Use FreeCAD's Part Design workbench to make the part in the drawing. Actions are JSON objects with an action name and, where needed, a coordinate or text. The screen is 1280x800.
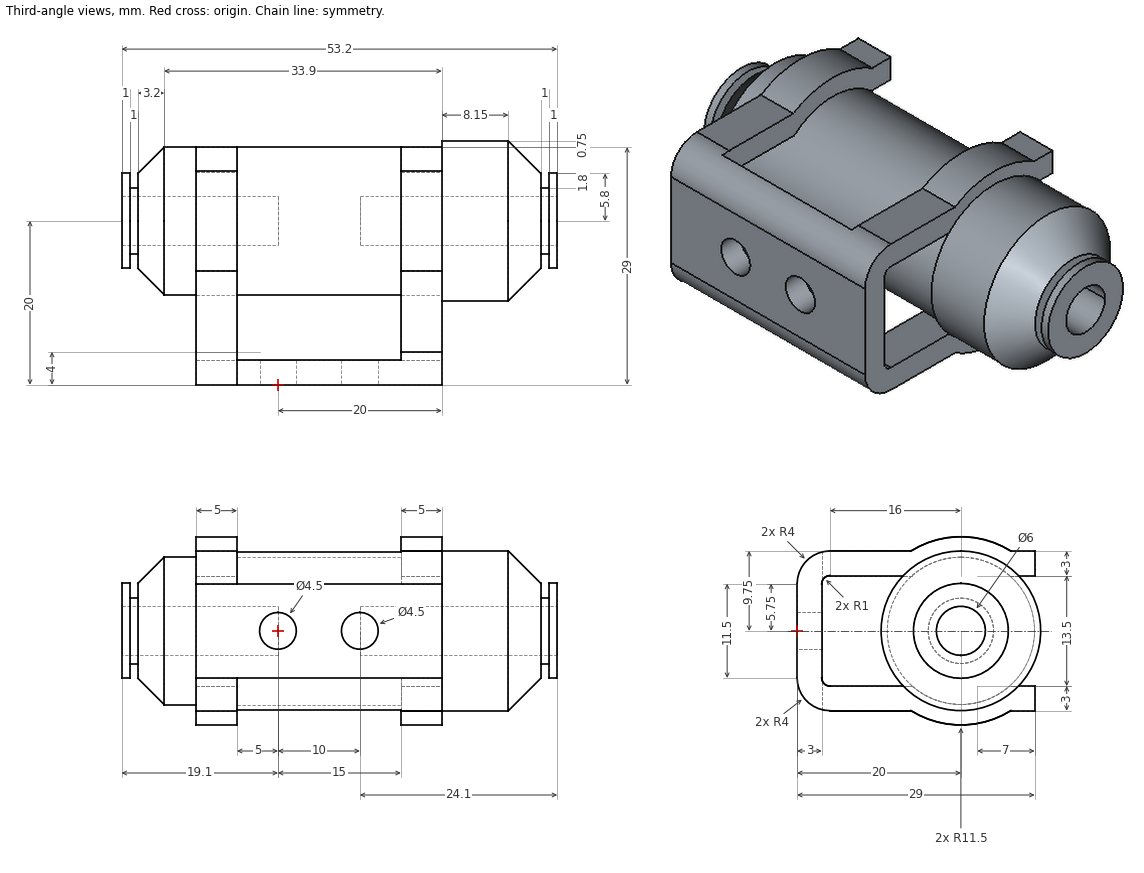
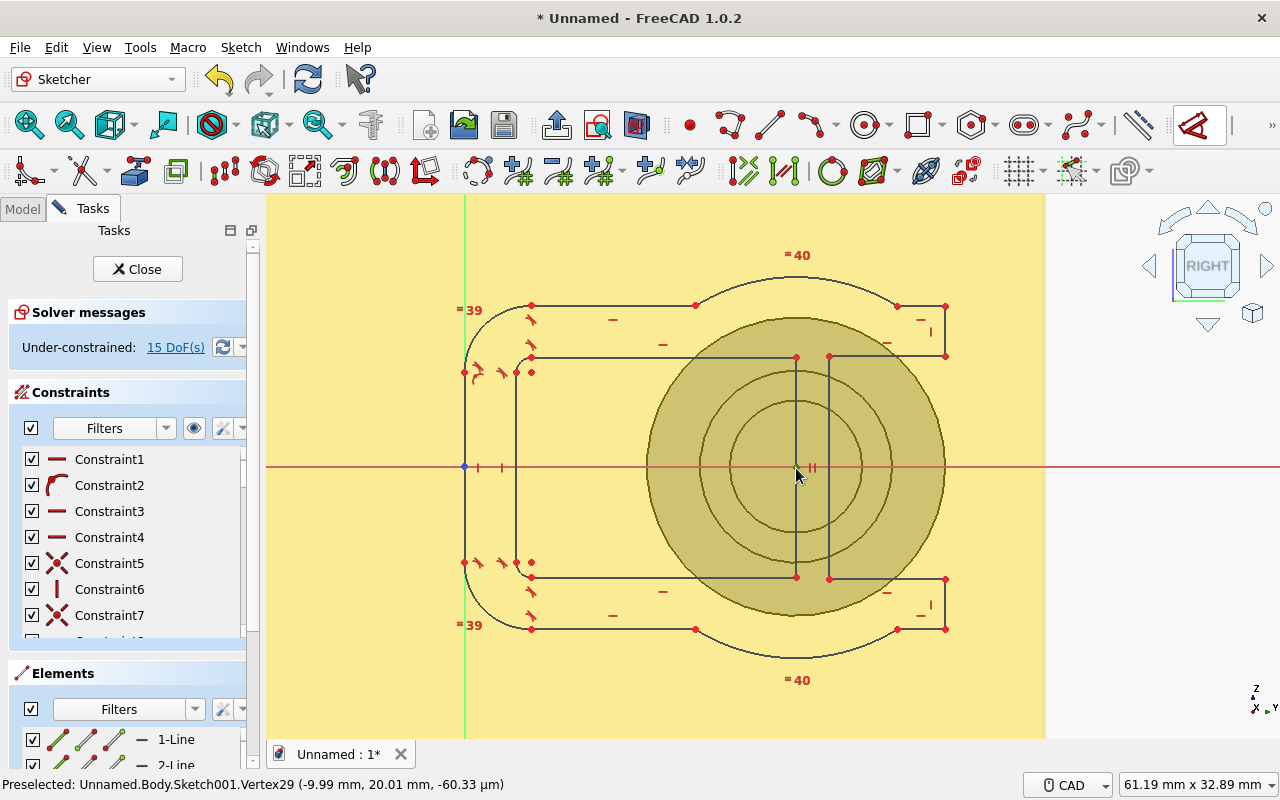
{"action": "left_click", "coordinate": [353, 467]}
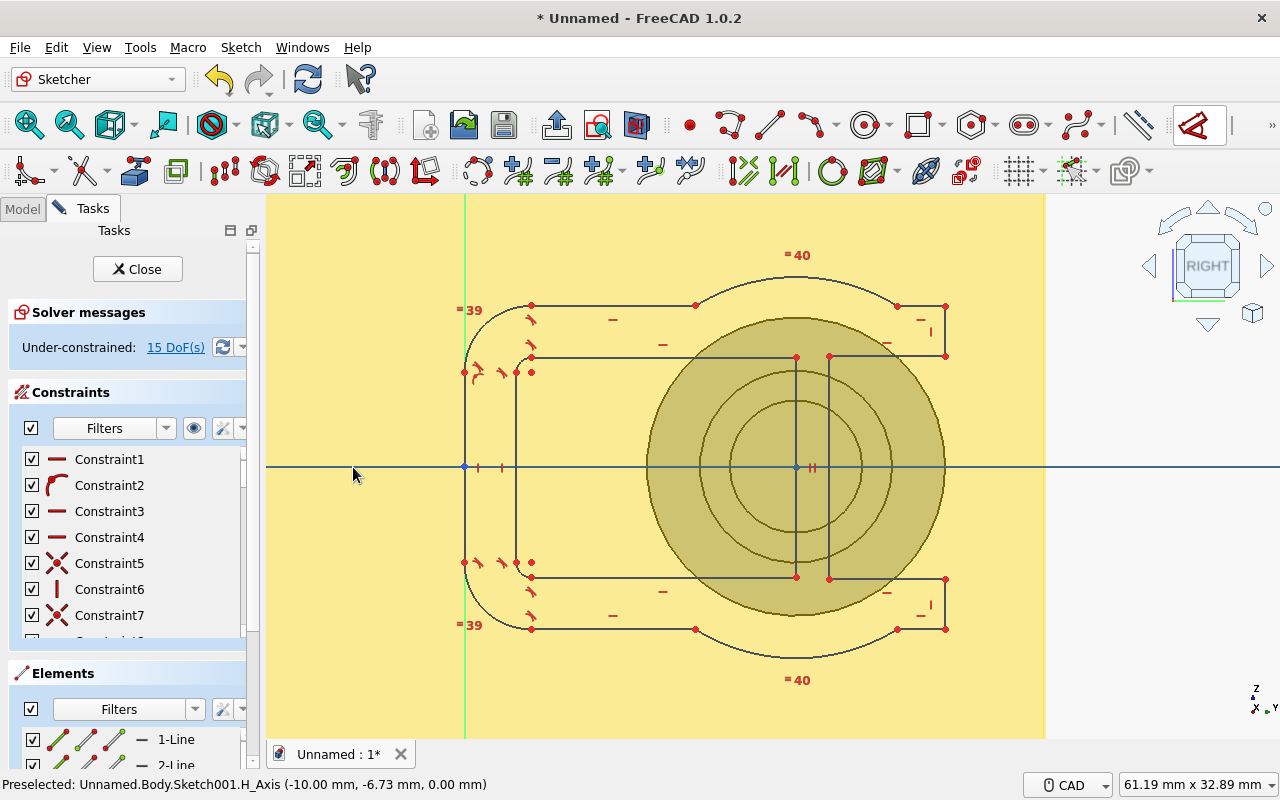
{"action": "key", "text": "c"}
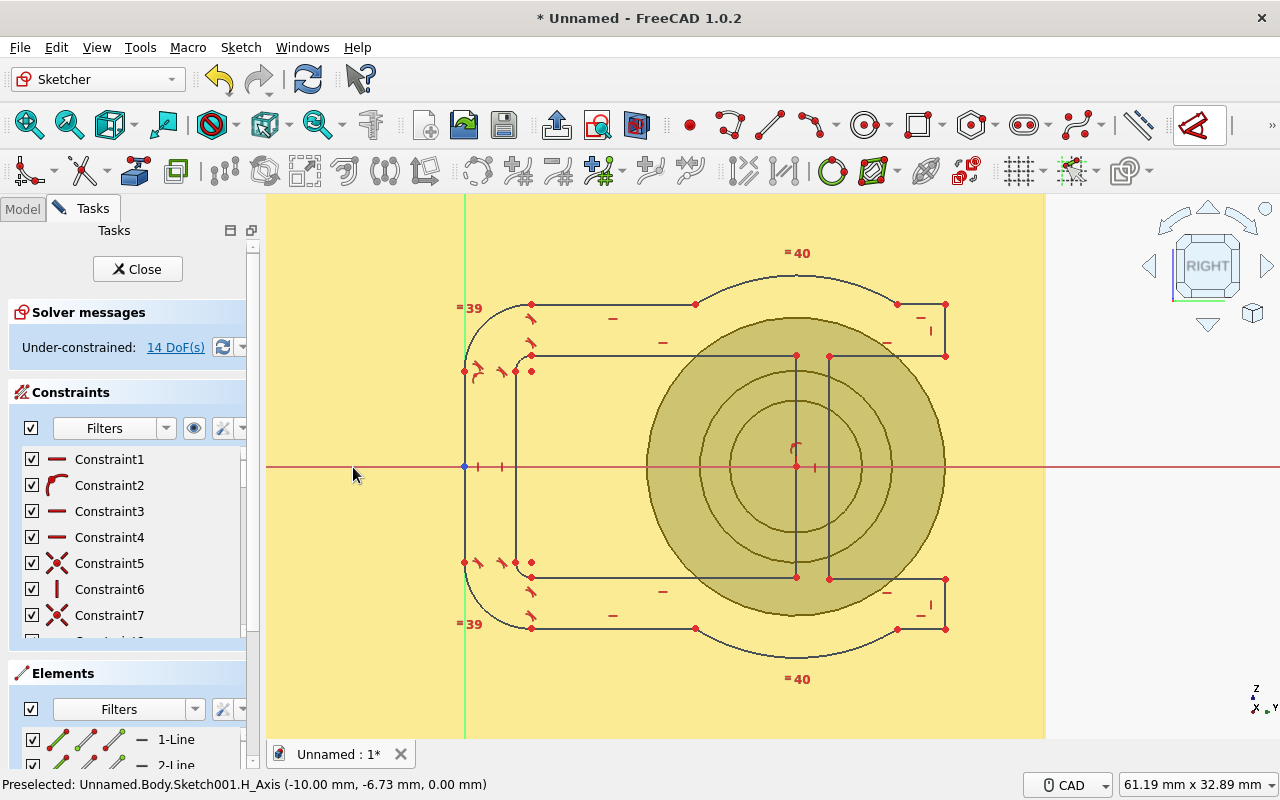
{"action": "left_click", "coordinate": [945, 579]}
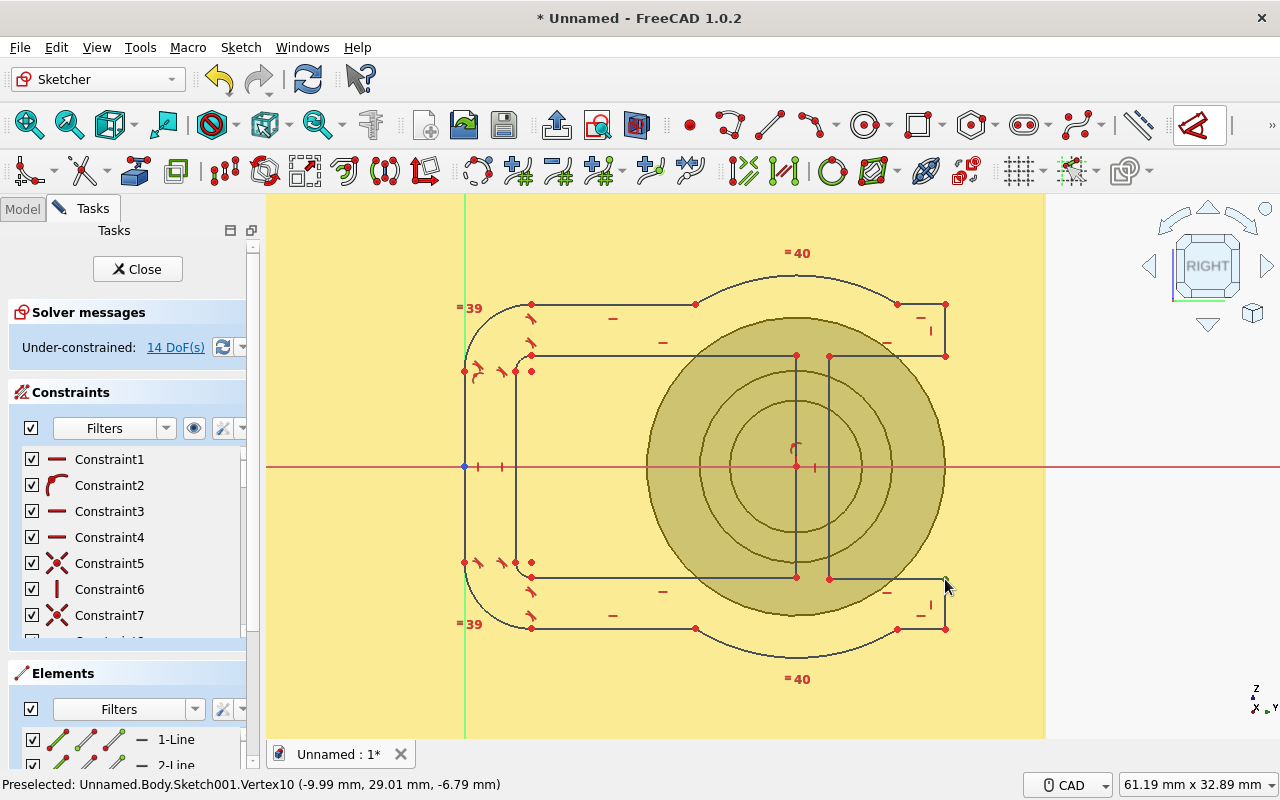
{"action": "left_click", "coordinate": [945, 356]}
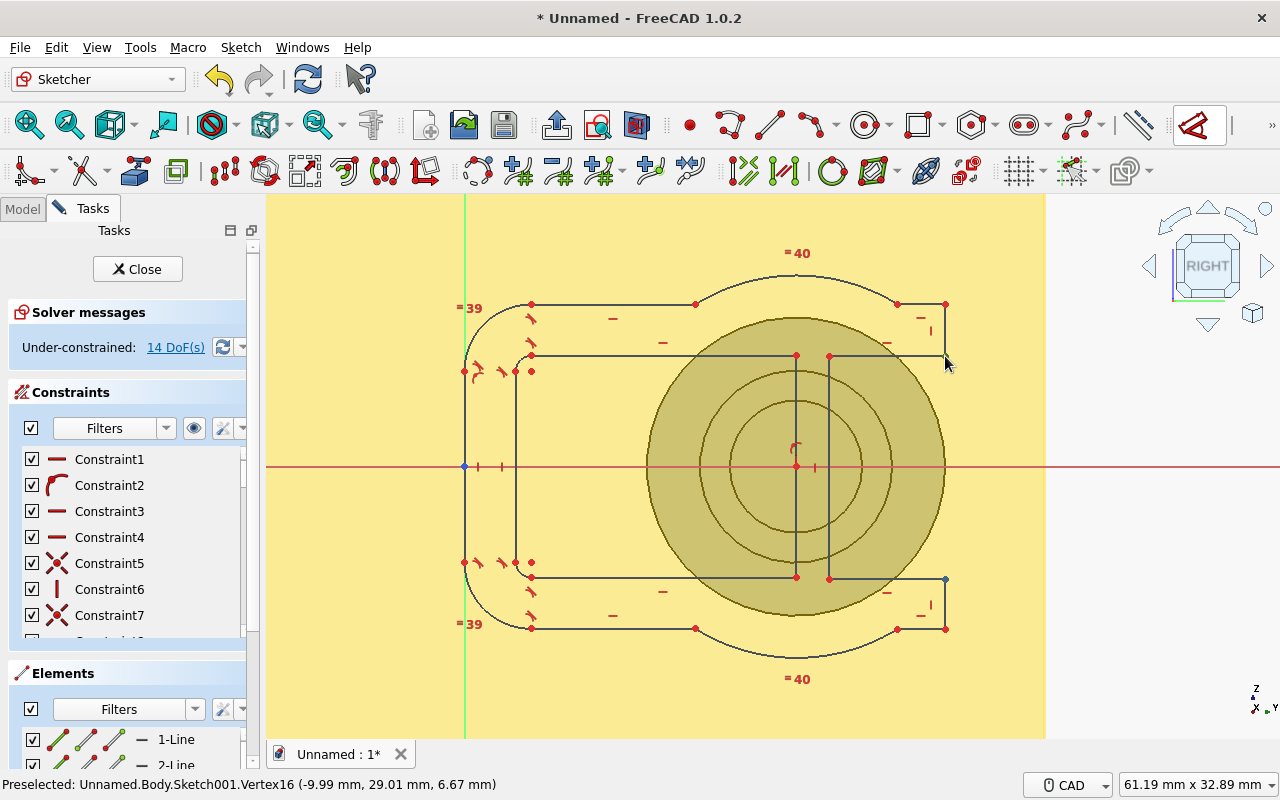
{"action": "left_click", "coordinate": [353, 467]}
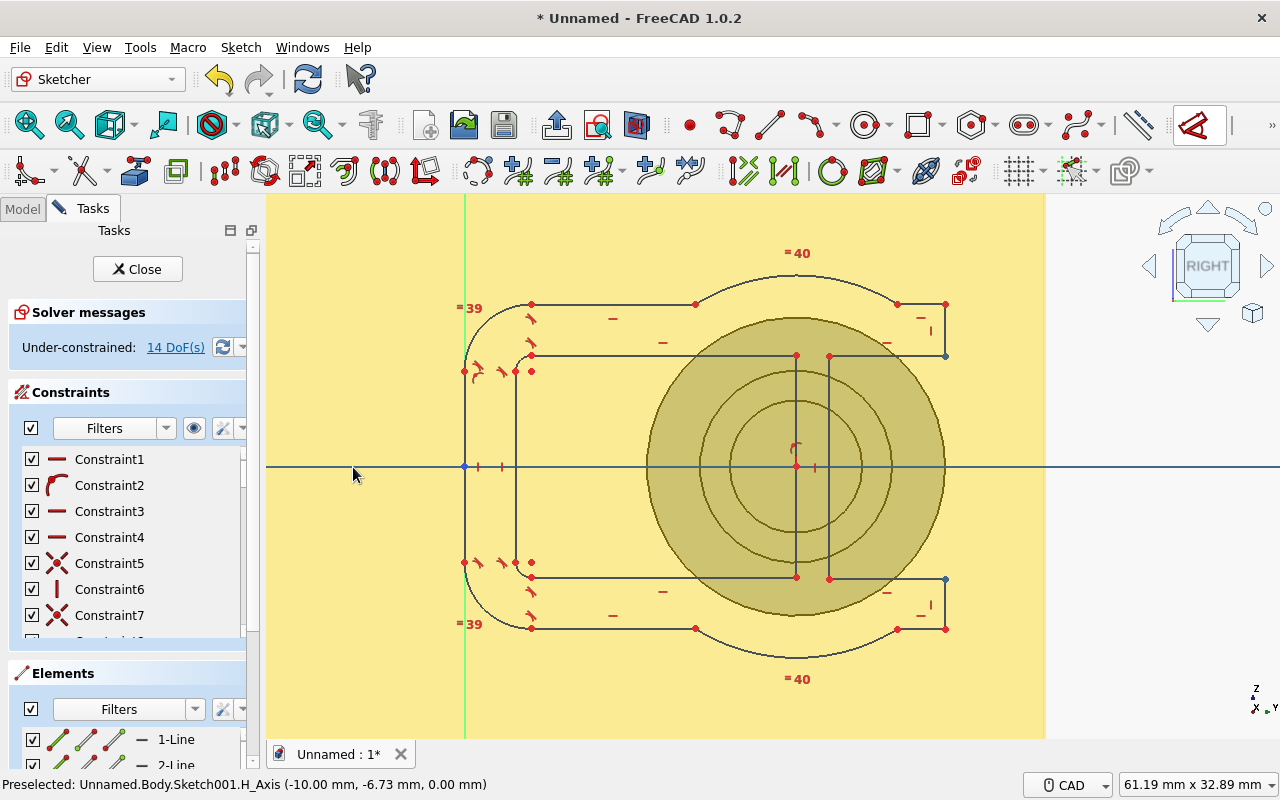
{"action": "key", "text": "s"}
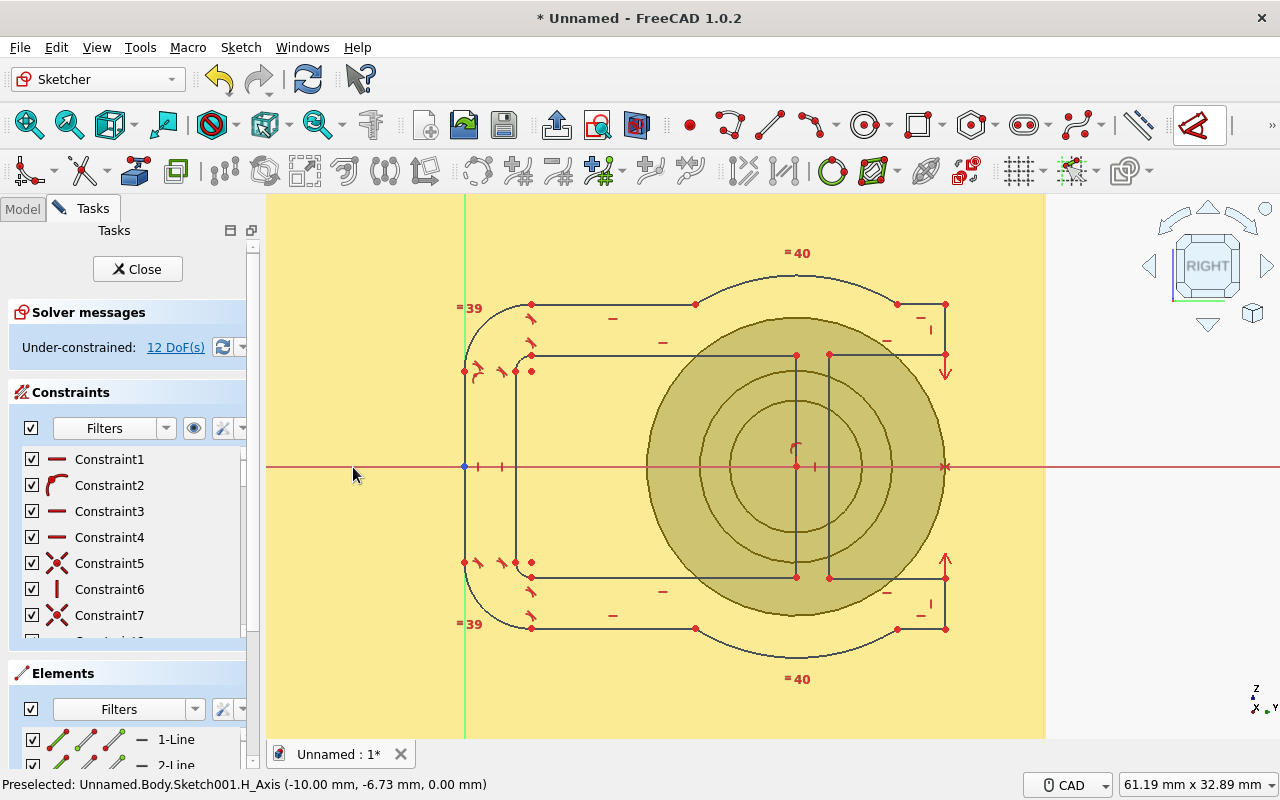
{"action": "left_click", "coordinate": [501, 312]}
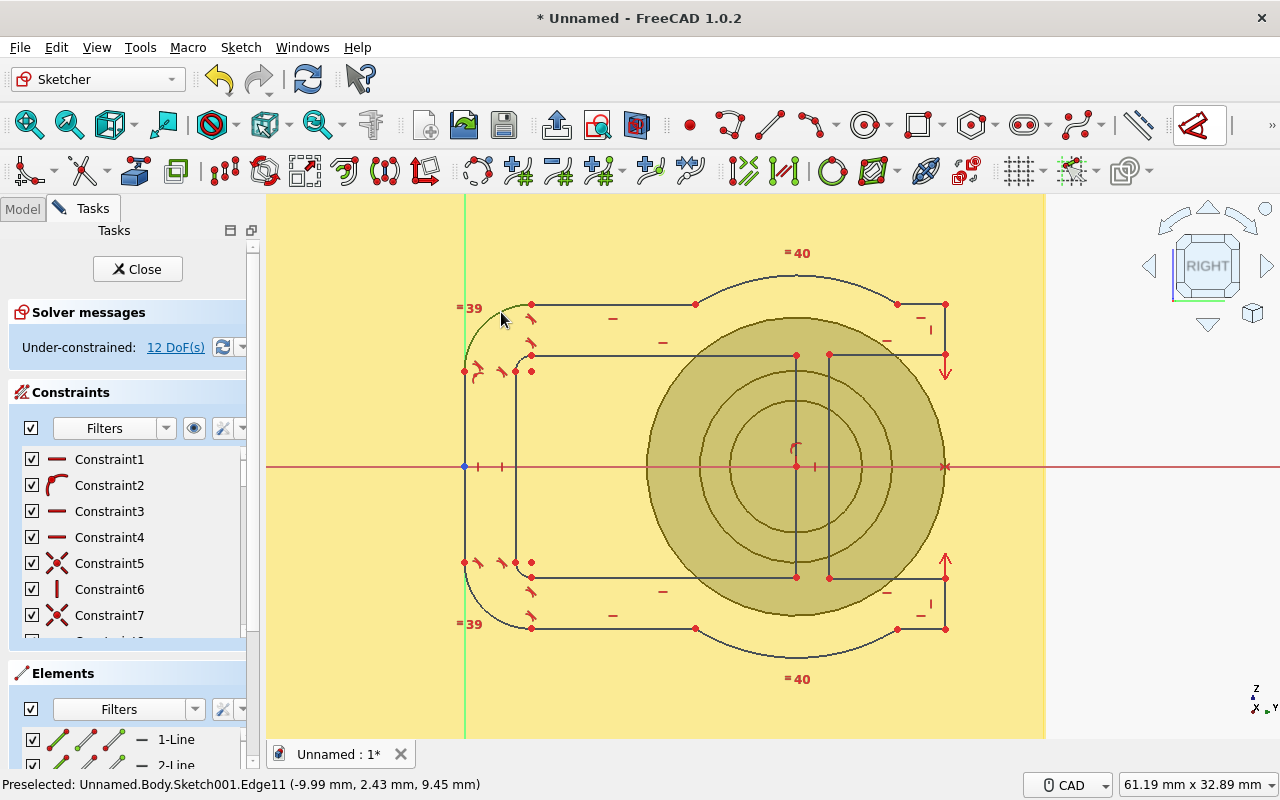
{"action": "key", "text": "k r"}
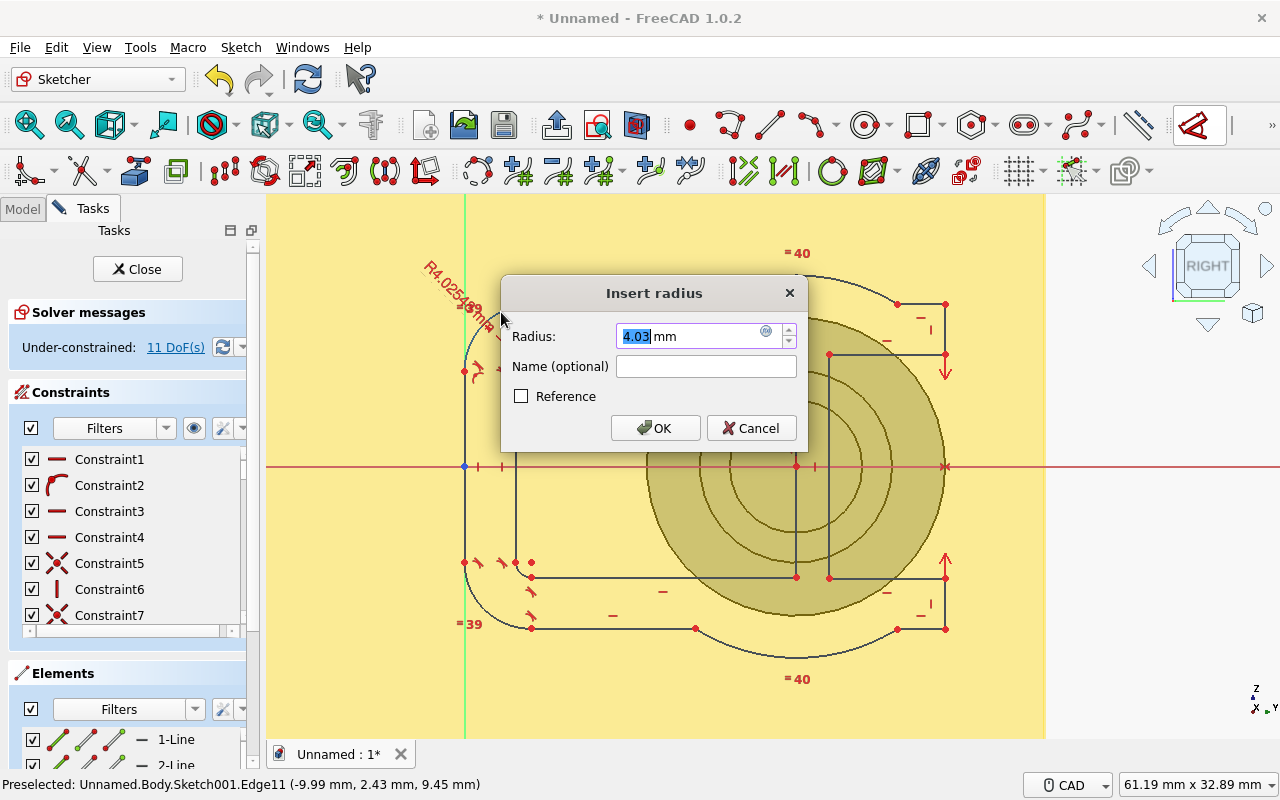
{"action": "type", "text": "4"}
{"action": "key", "text": "Return"}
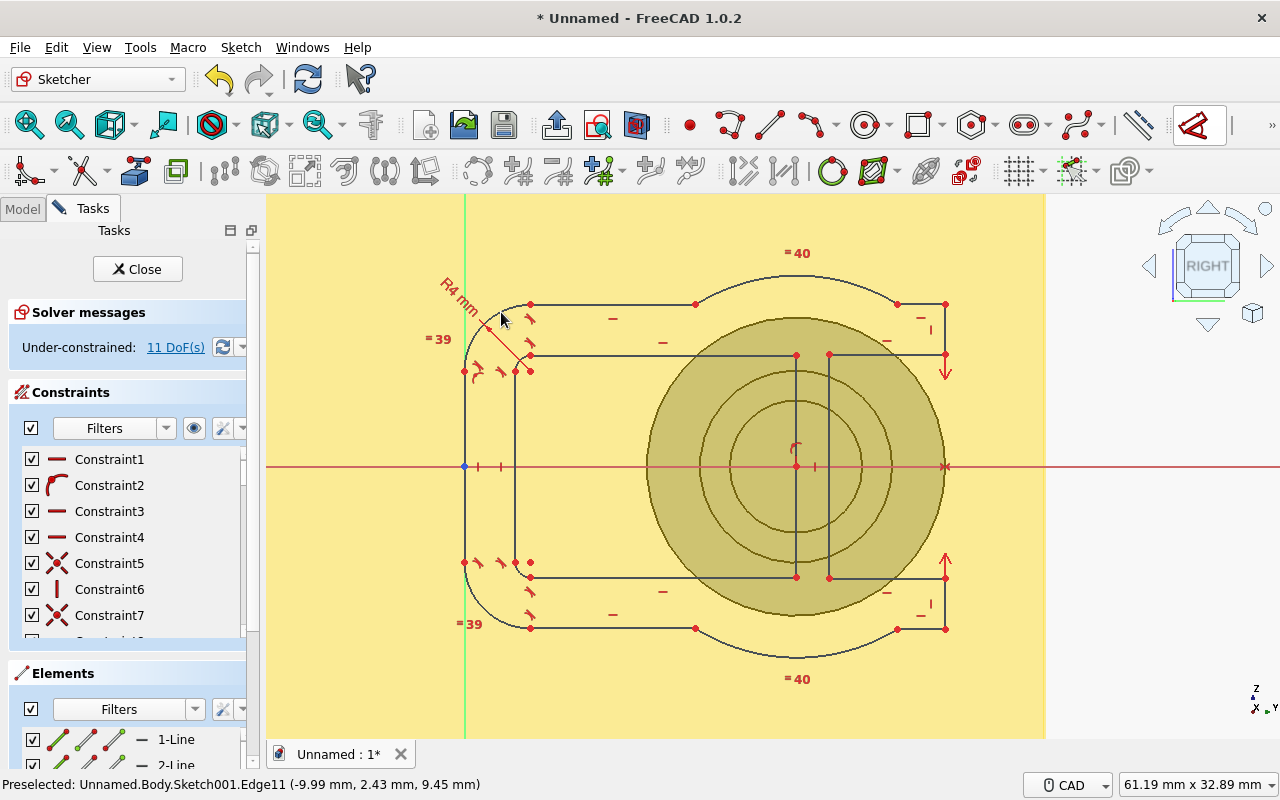
{"action": "left_click", "coordinate": [754, 653]}